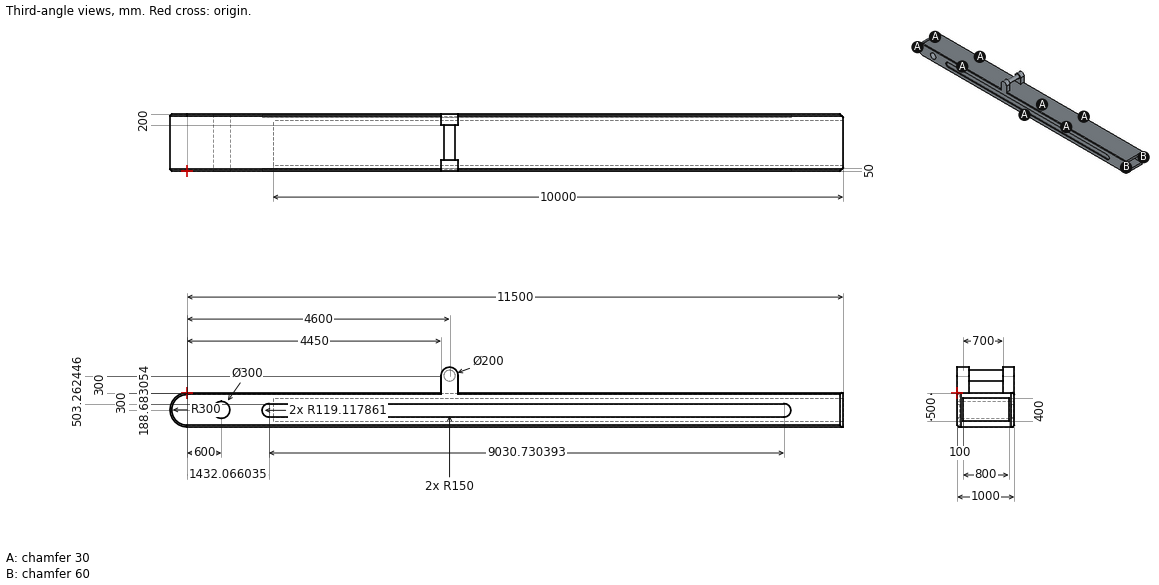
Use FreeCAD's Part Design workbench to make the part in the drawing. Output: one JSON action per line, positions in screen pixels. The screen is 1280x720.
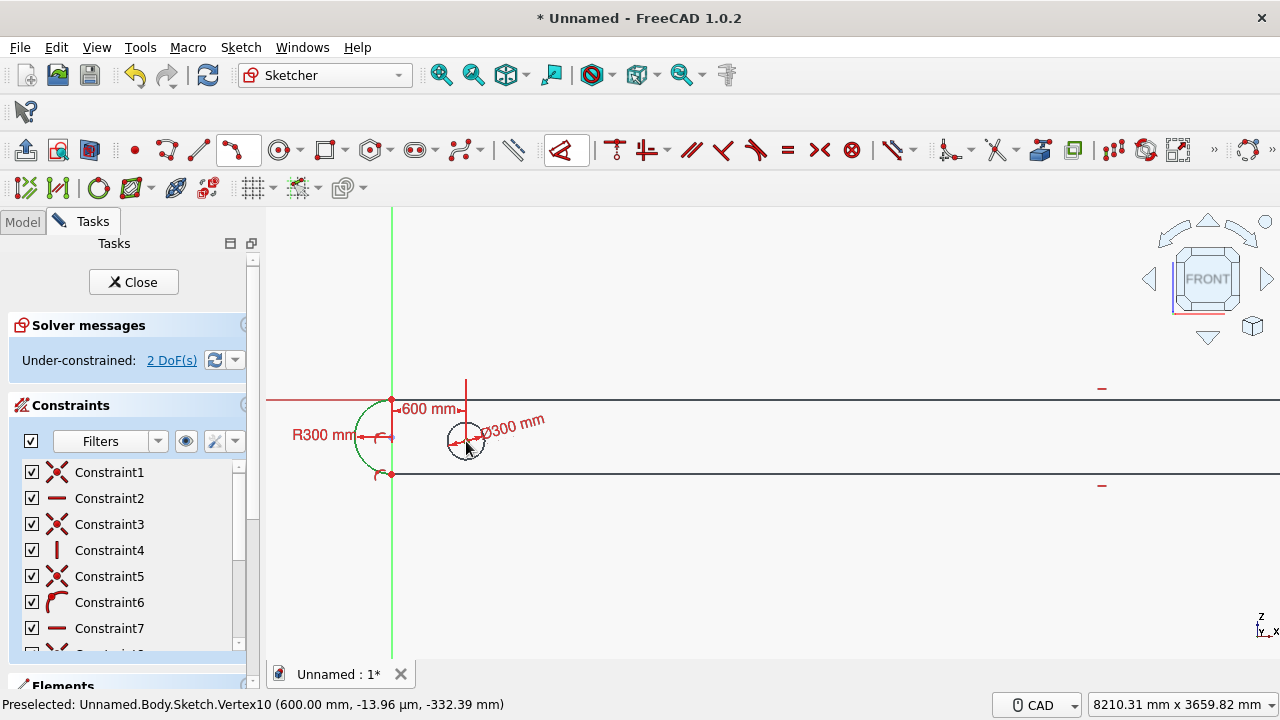
{"action": "key", "text": "i"}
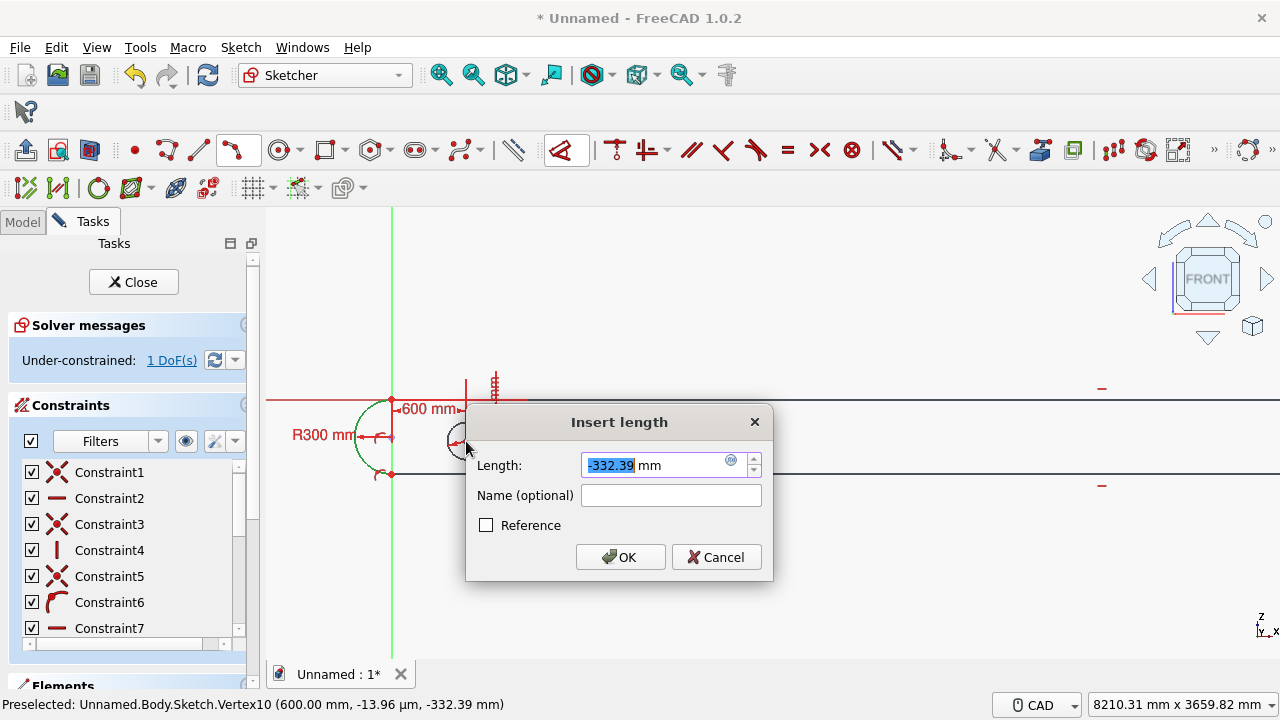
{"action": "type", "text": "-300"}
{"action": "key", "text": "Return"}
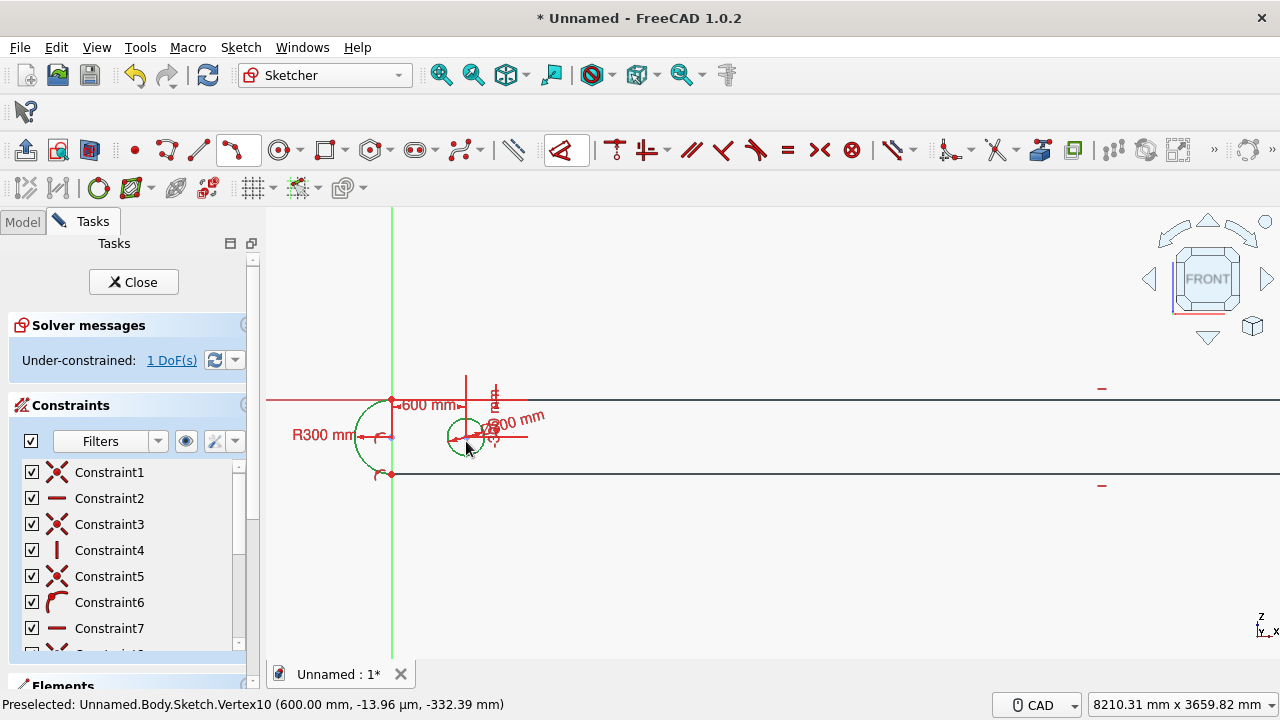
{"action": "left_click", "coordinate": [818, 400]}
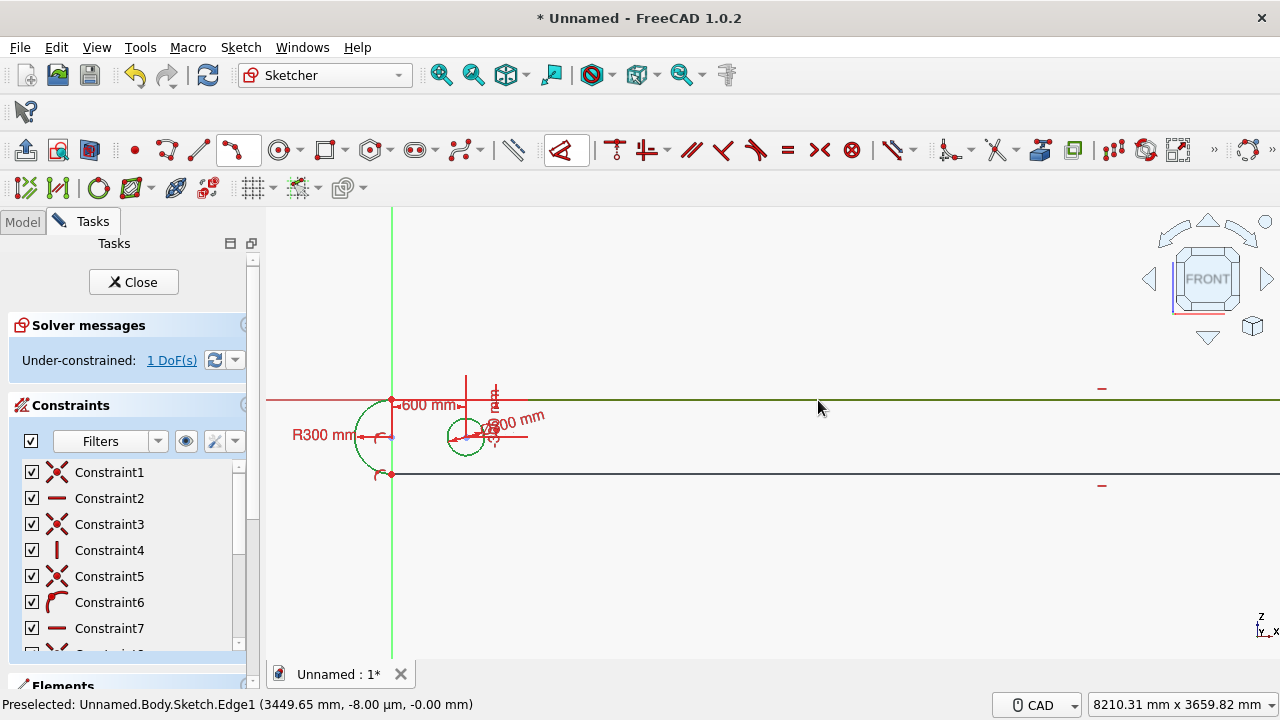
{"action": "key", "text": "l"}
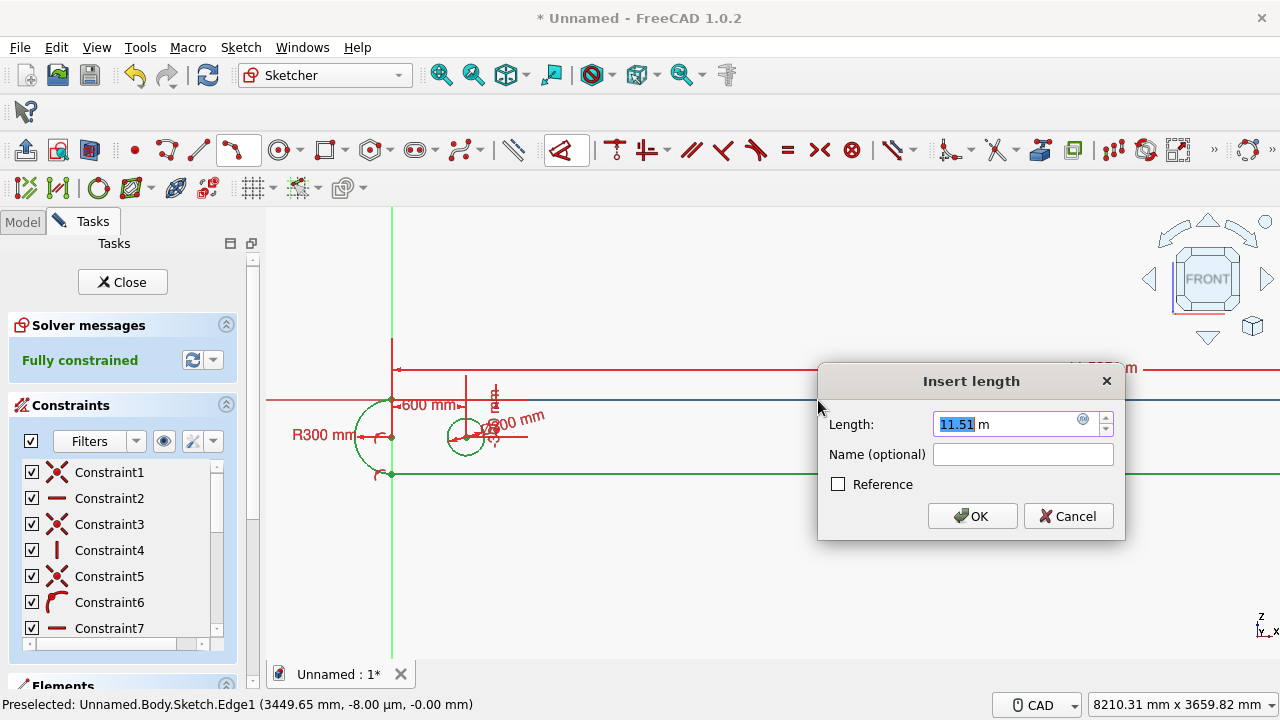
{"action": "key", "text": "ctrl+a"}
{"action": "type", "text": "11500 mm"}
{"action": "key", "text": "Return"}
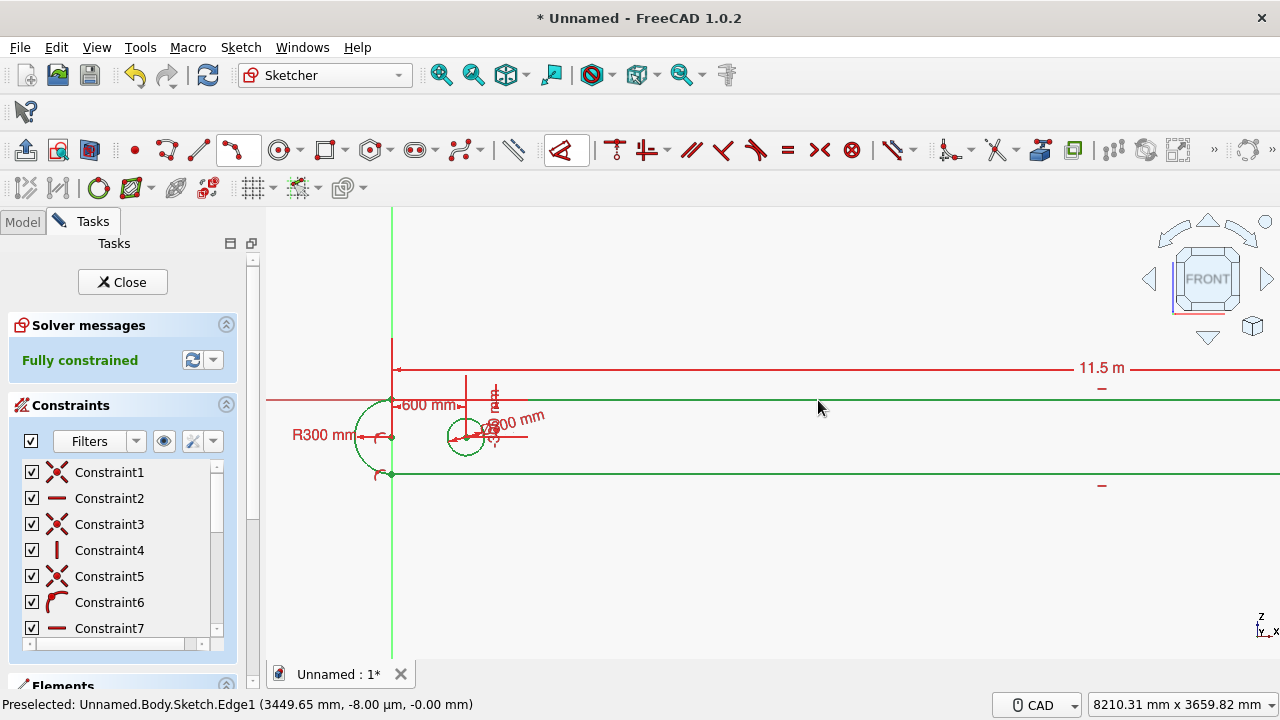
{"action": "left_click", "coordinate": [123, 282]}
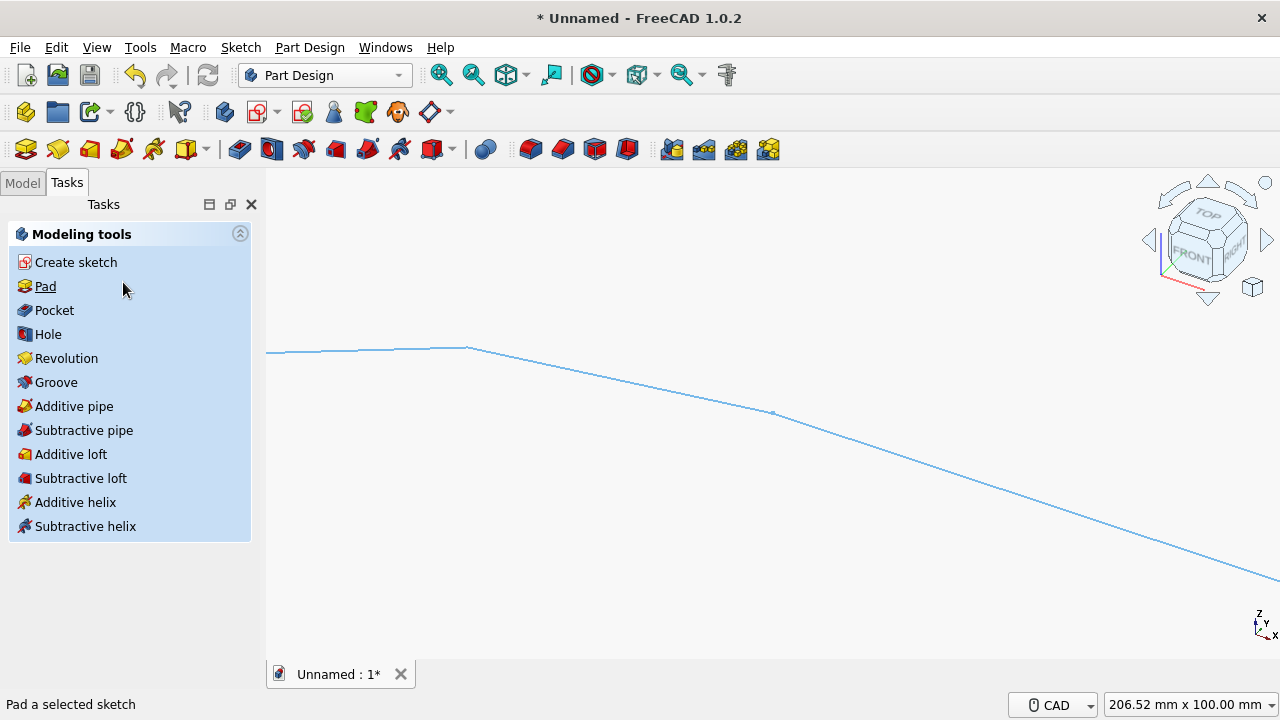
{"action": "left_click", "coordinate": [26, 150]}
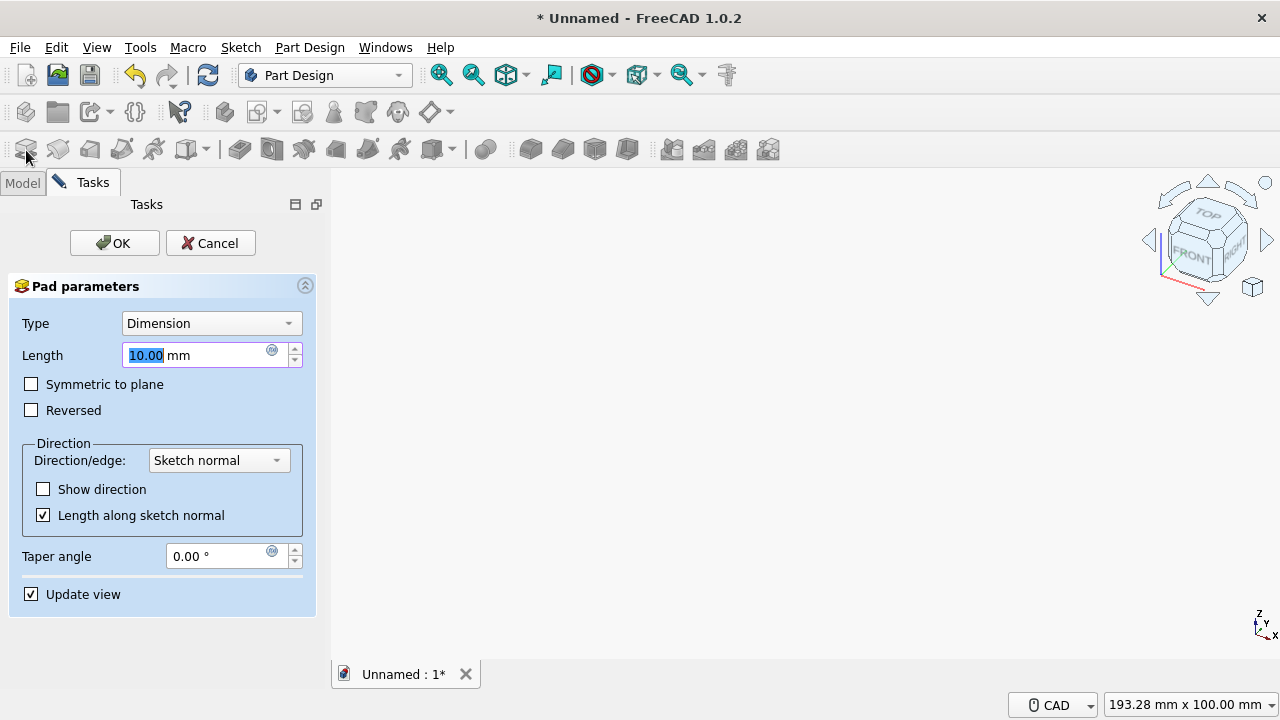
{"action": "type", "text": "1000"}
{"action": "key", "text": "Tab"}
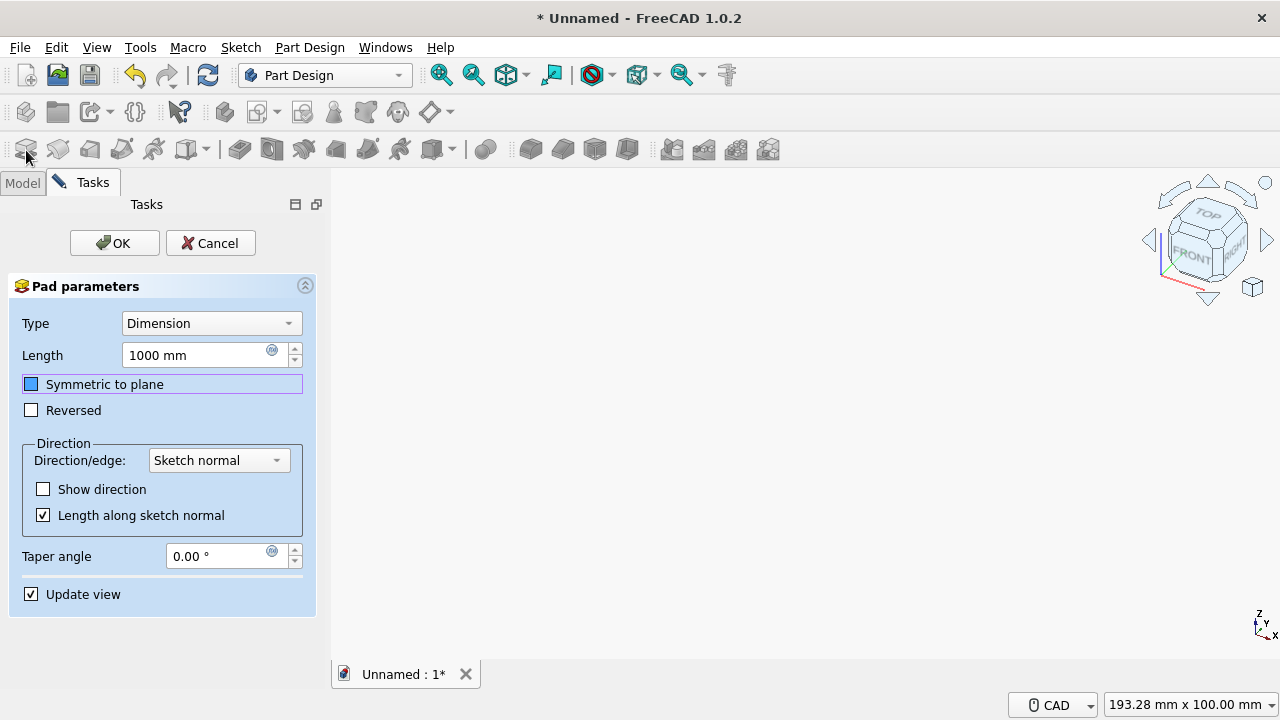
{"action": "left_click", "coordinate": [30, 410]}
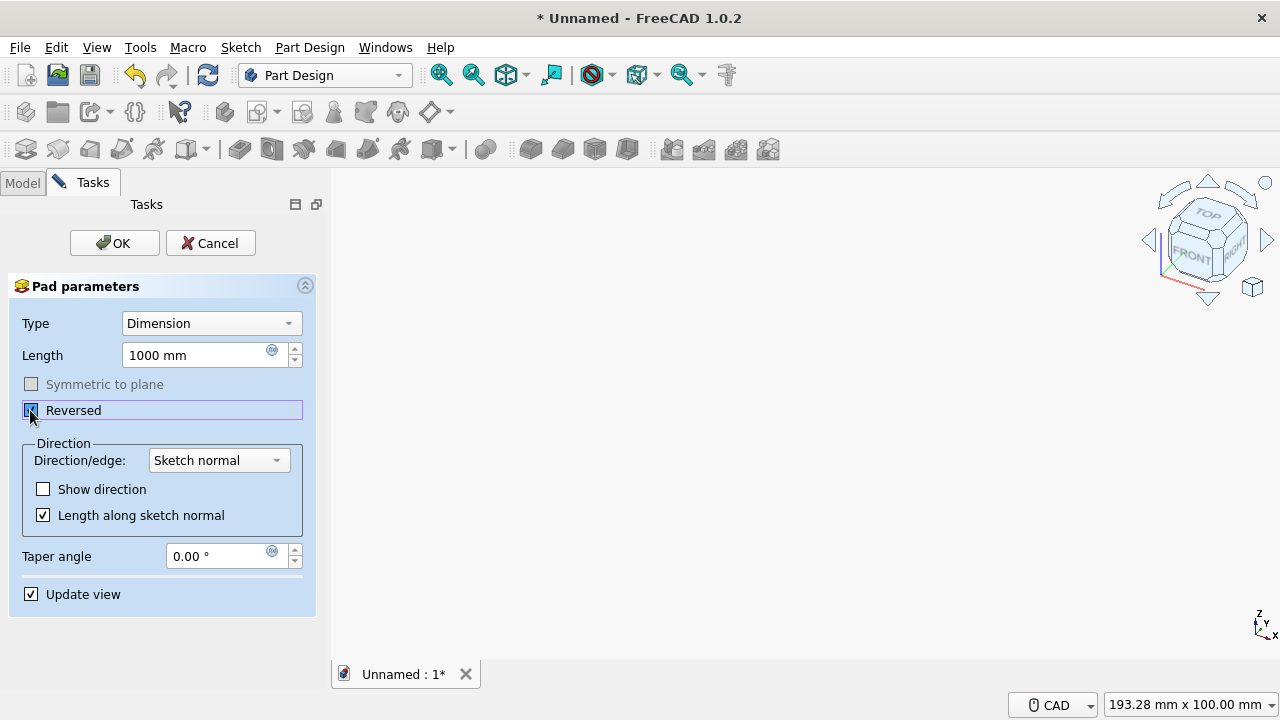
{"action": "left_click", "coordinate": [115, 243]}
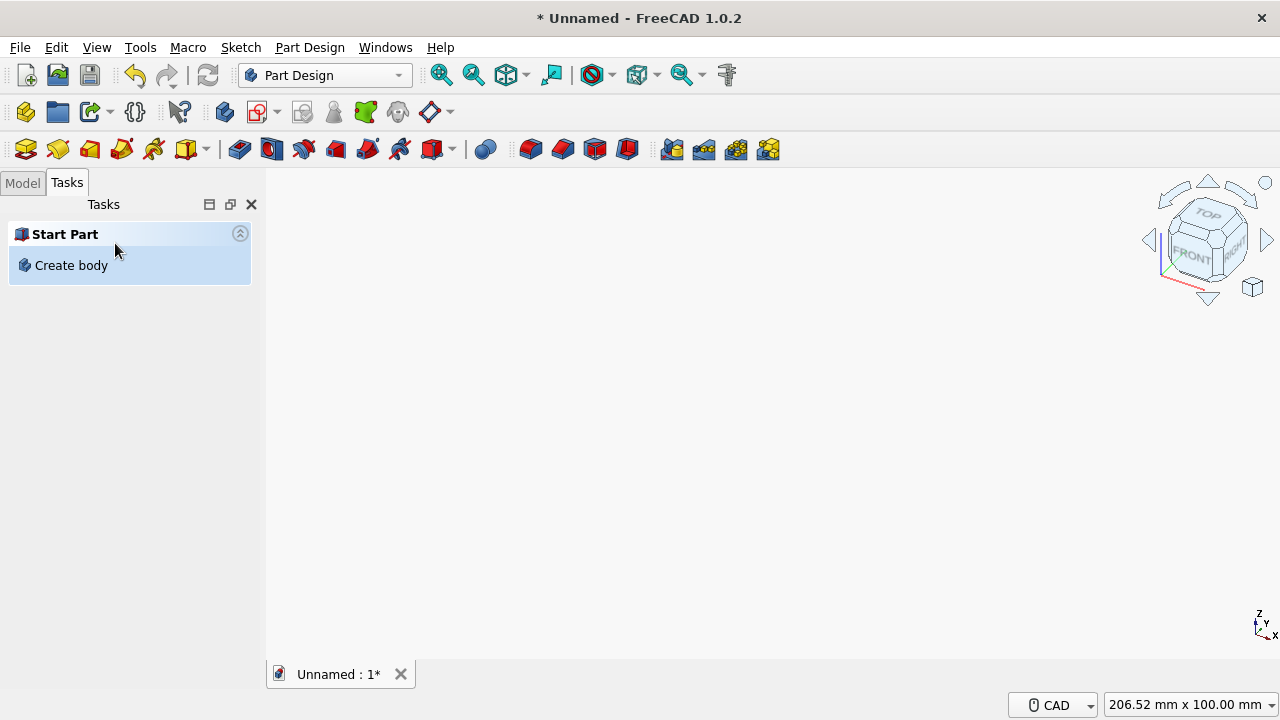
{"action": "left_click", "coordinate": [442, 76]}